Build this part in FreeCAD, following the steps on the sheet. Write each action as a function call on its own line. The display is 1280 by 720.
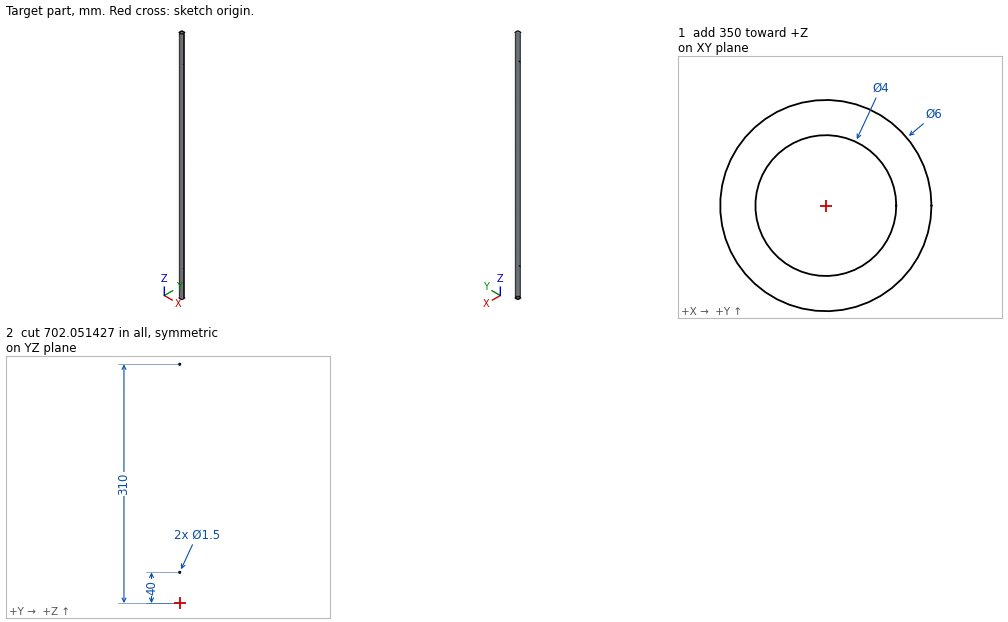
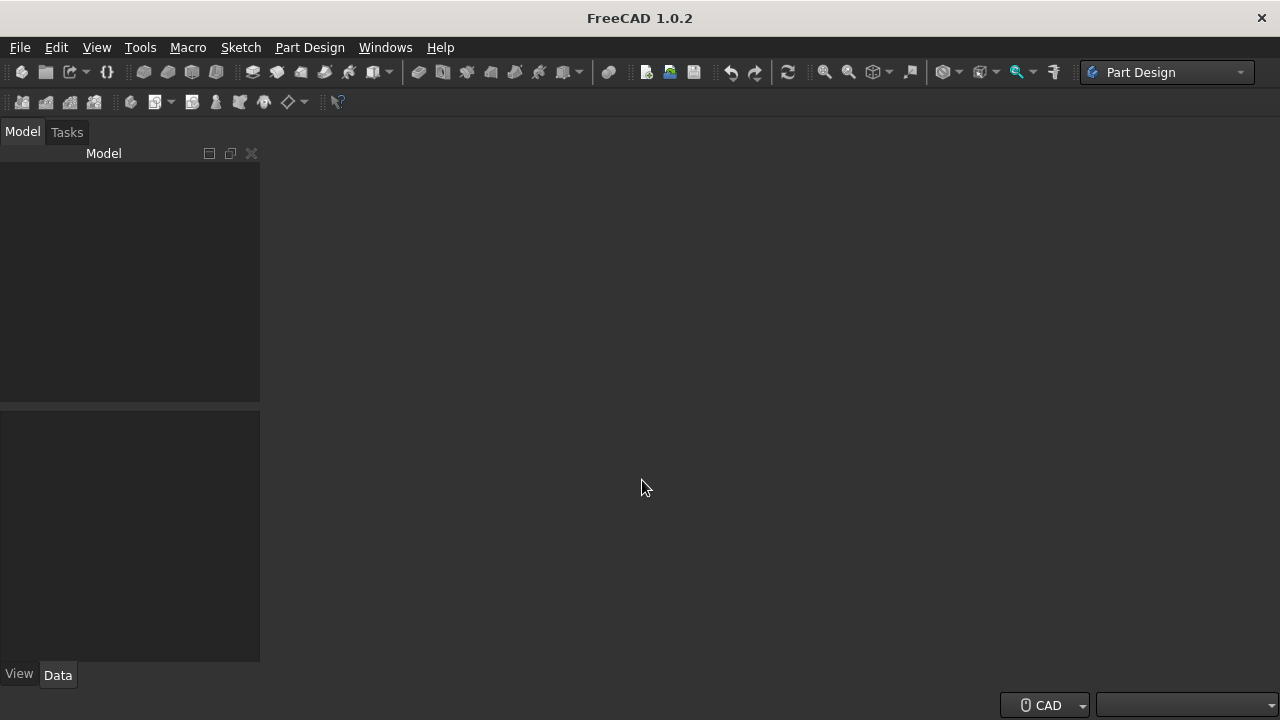
key(ctrl+n)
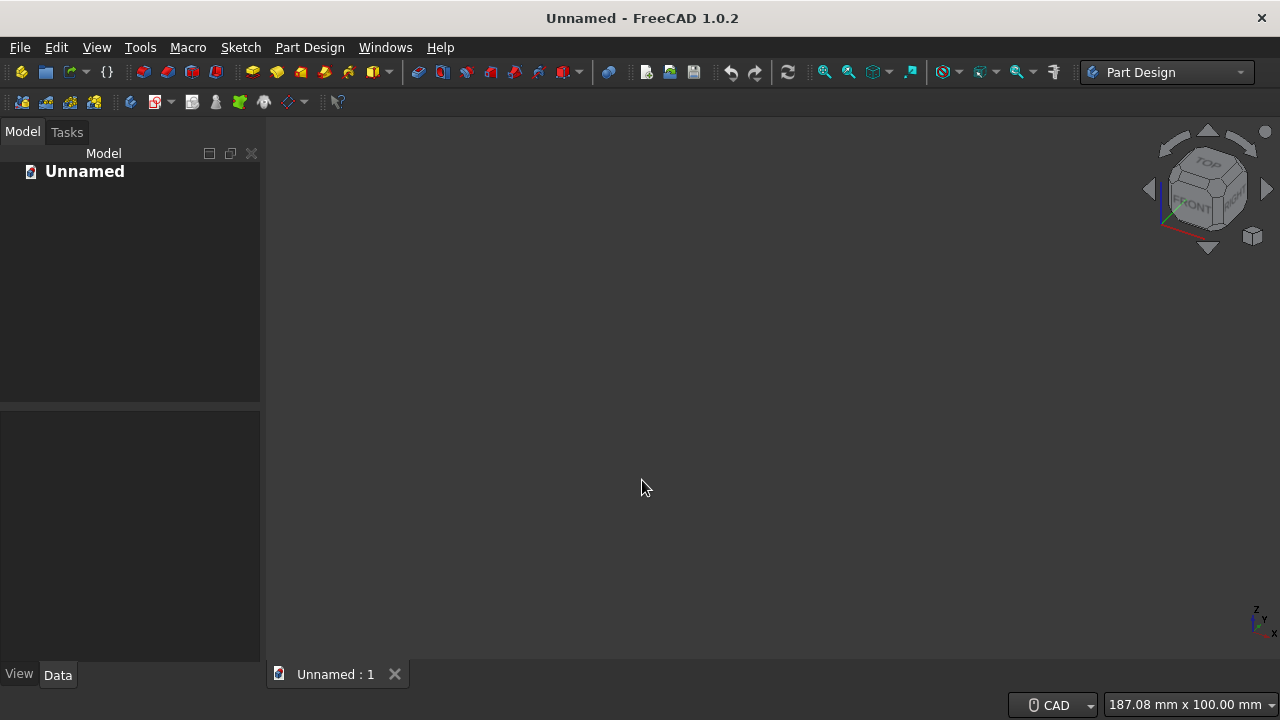
click(156, 102)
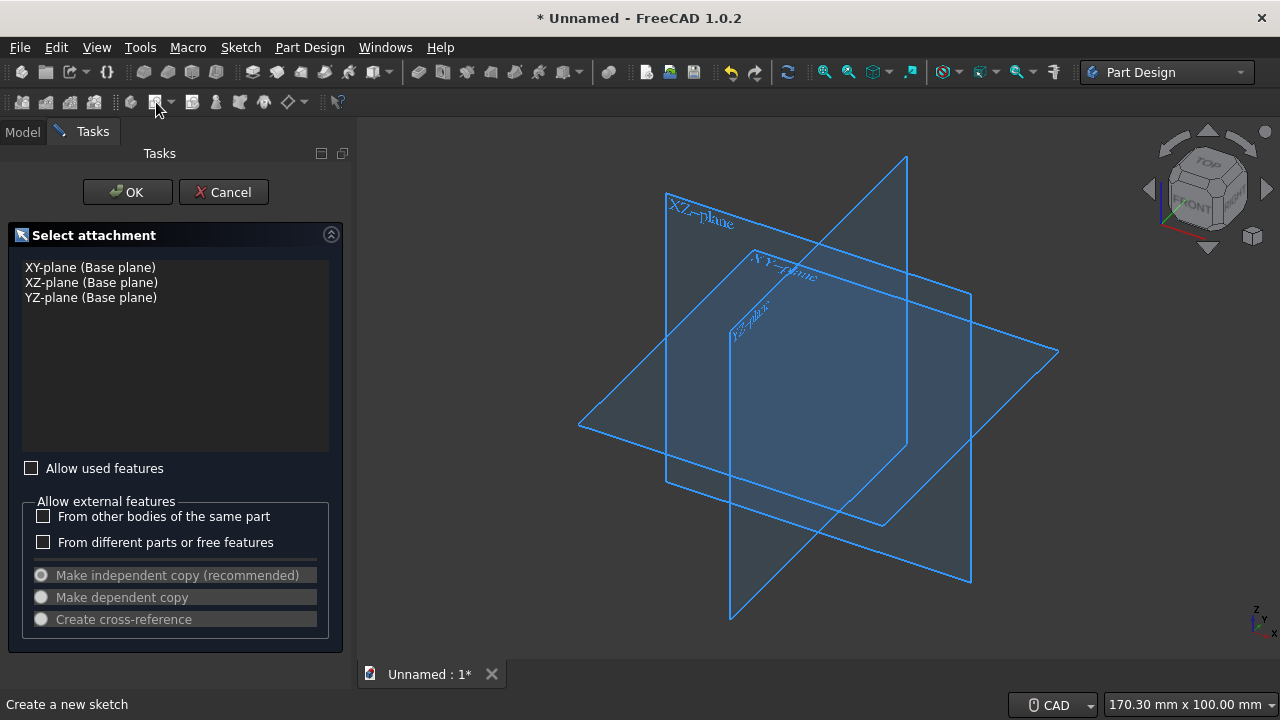
click(82, 268)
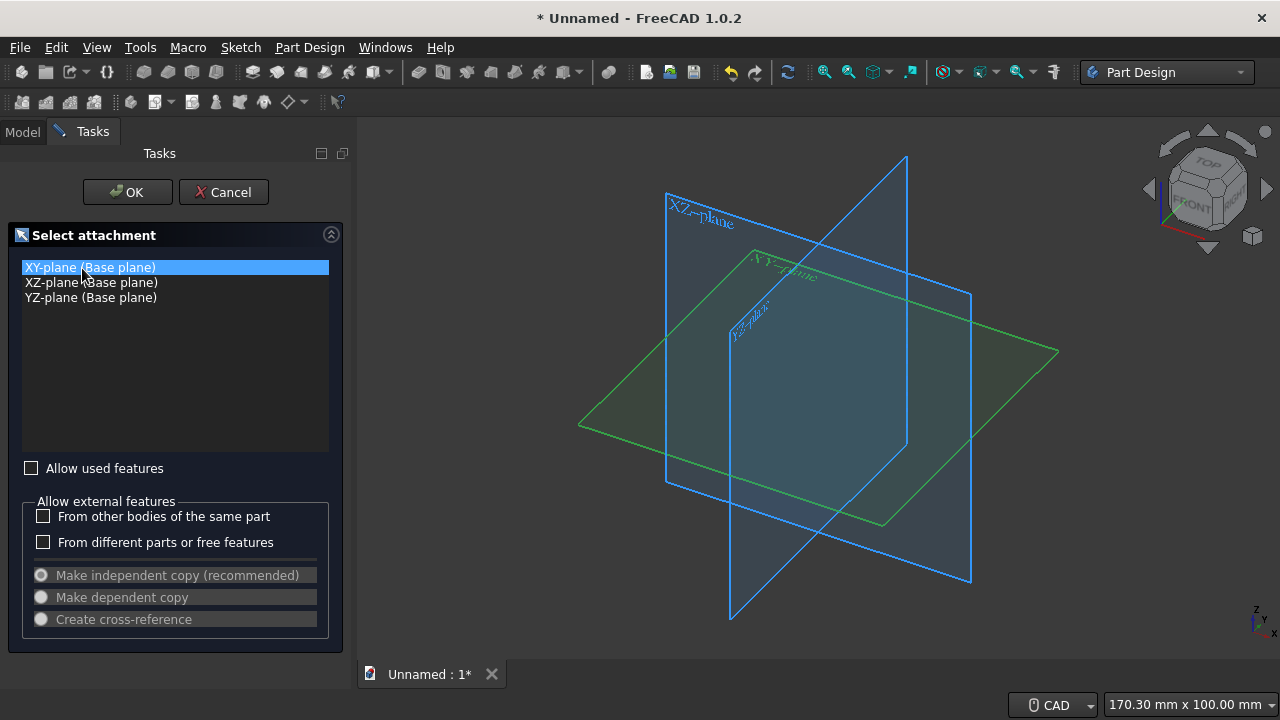
click(128, 192)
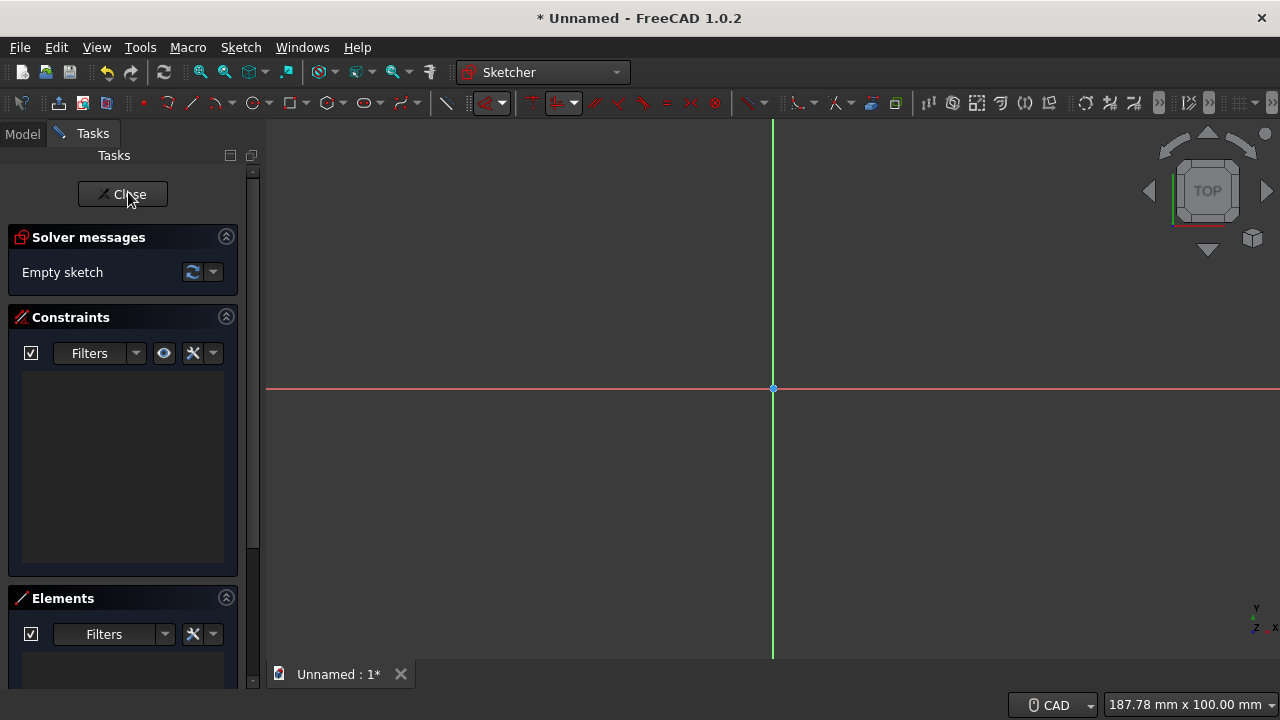
scroll(780, 389, up, 12)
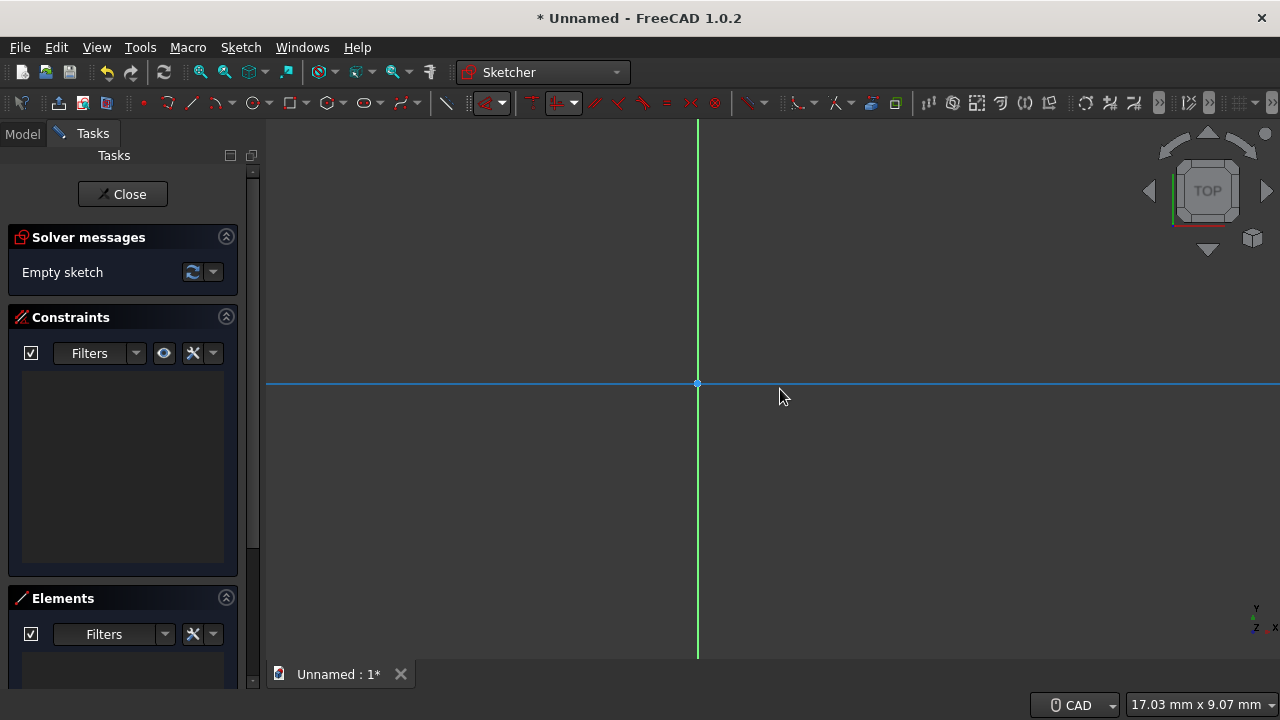
click(254, 104)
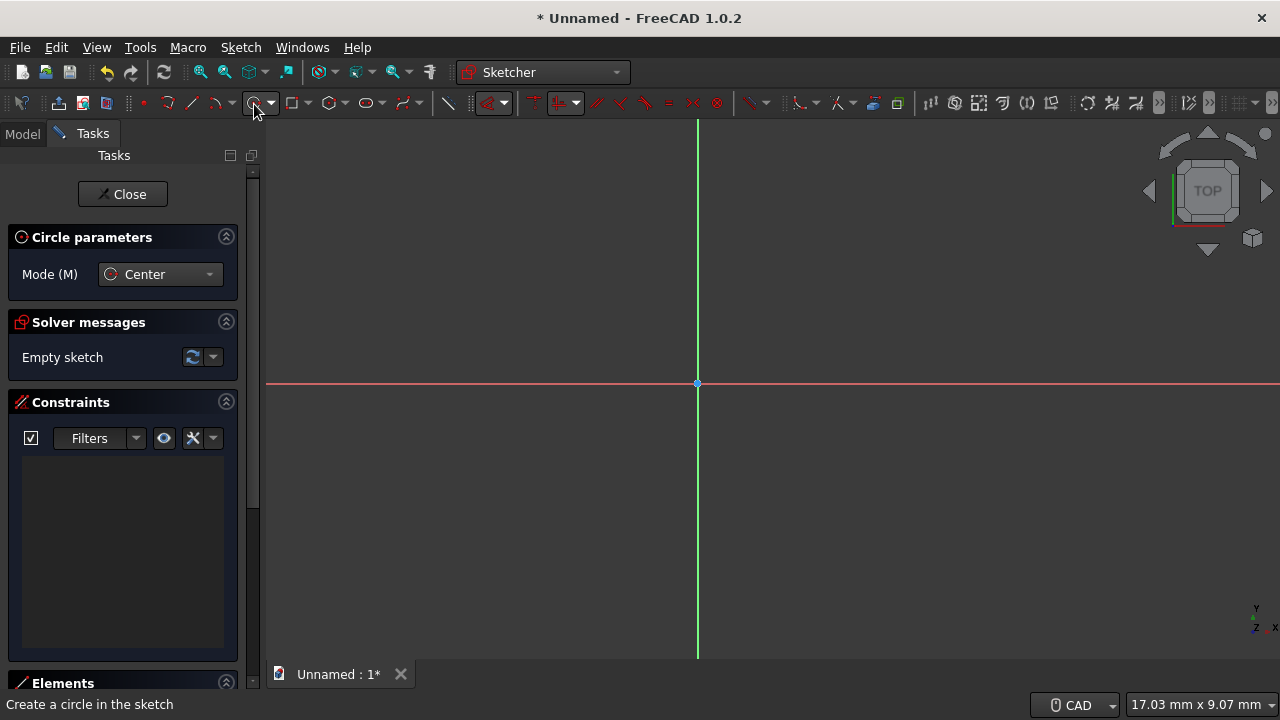
click(698, 384)
move(824, 258)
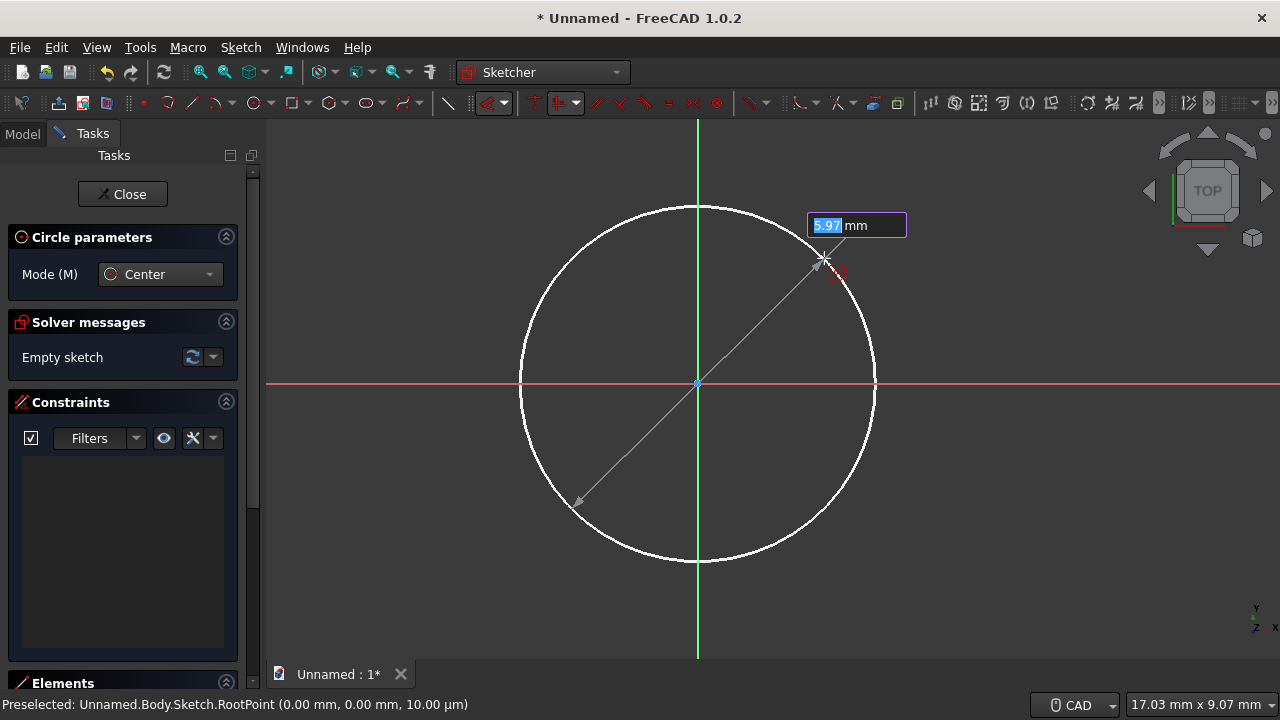
text(6)
key(Return)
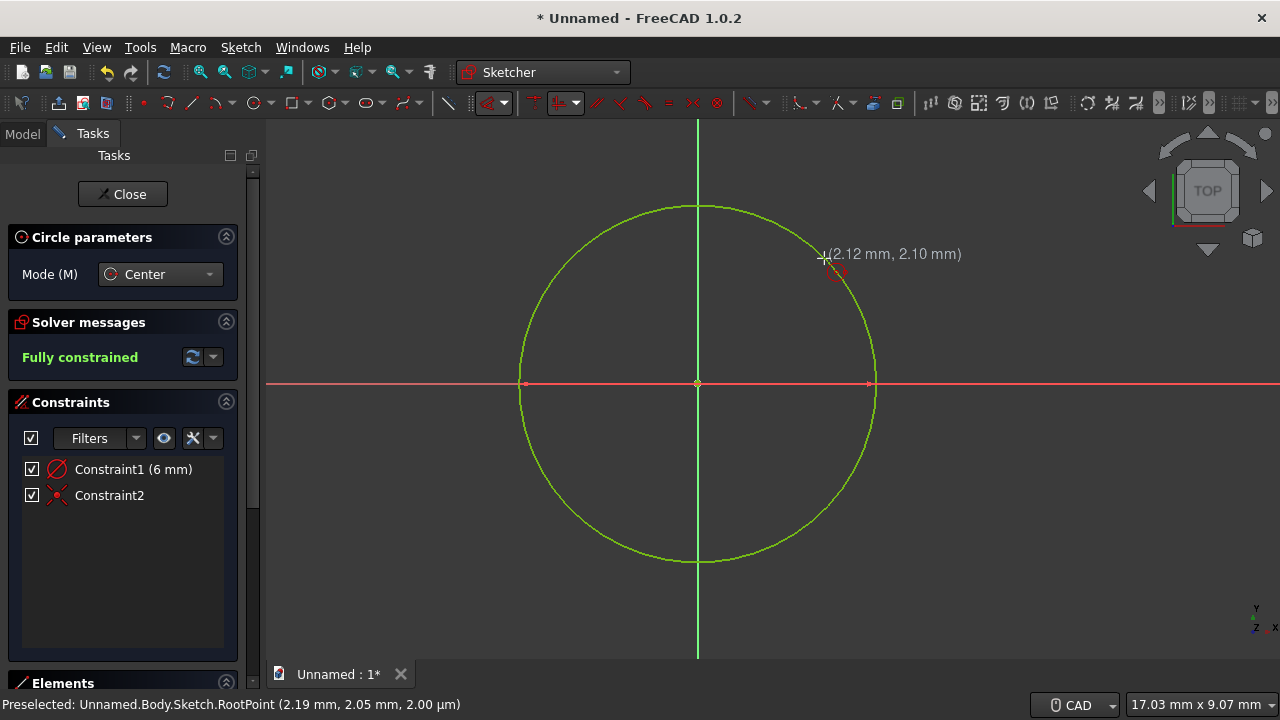
click(698, 384)
move(782, 300)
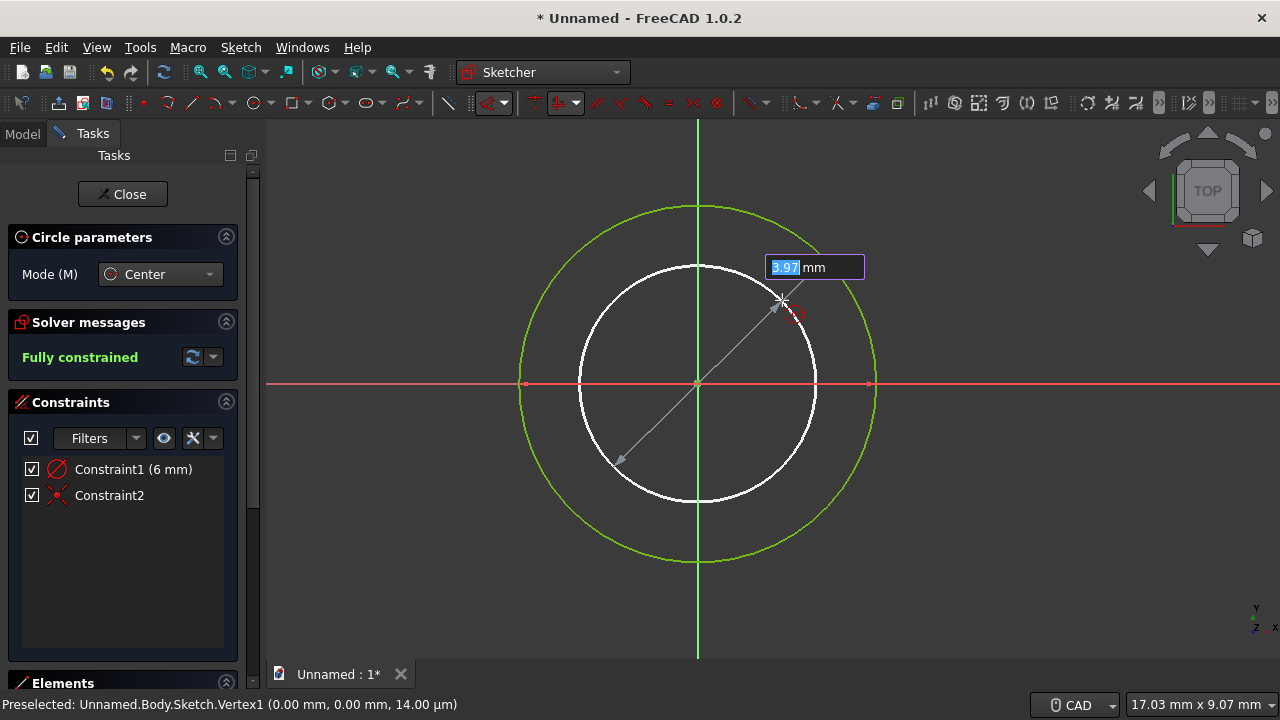
text(4)
key(Return)
key(Escape)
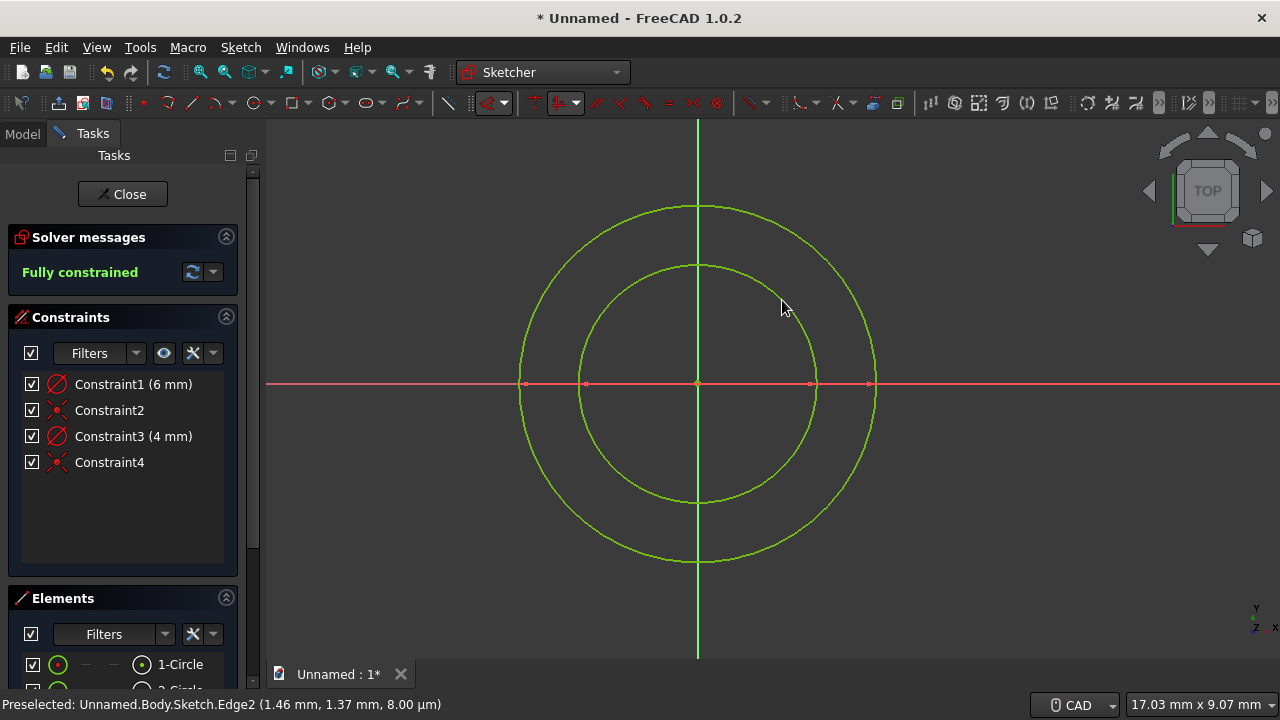
click(123, 194)